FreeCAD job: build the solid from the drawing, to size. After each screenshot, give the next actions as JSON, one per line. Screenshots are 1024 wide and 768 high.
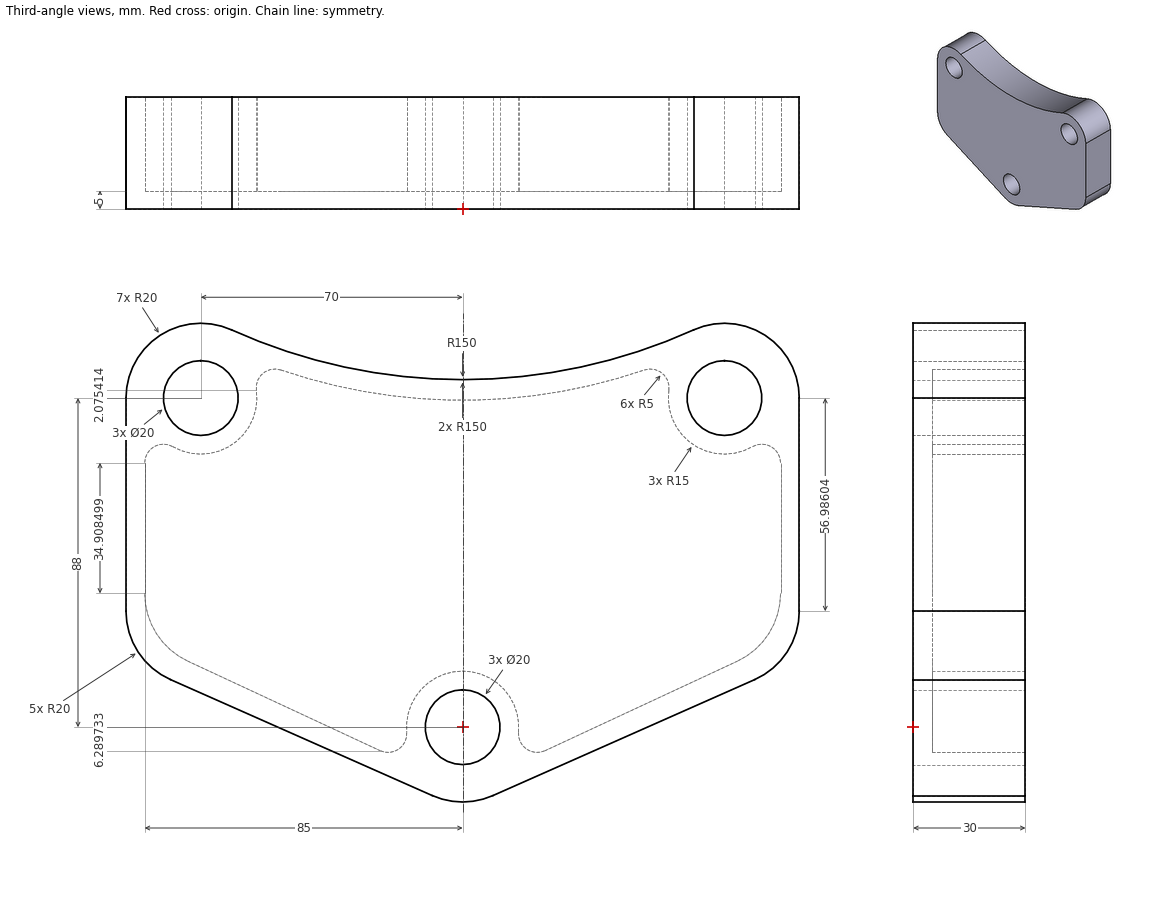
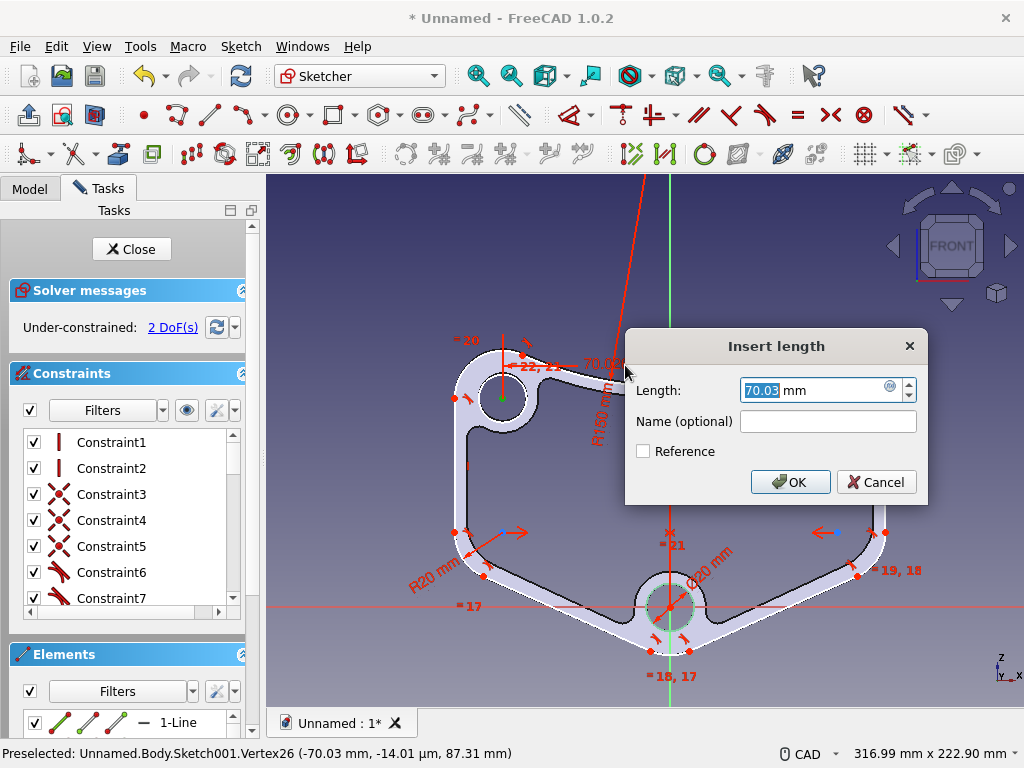
{"action": "type", "text": "70"}
{"action": "key", "text": "Return"}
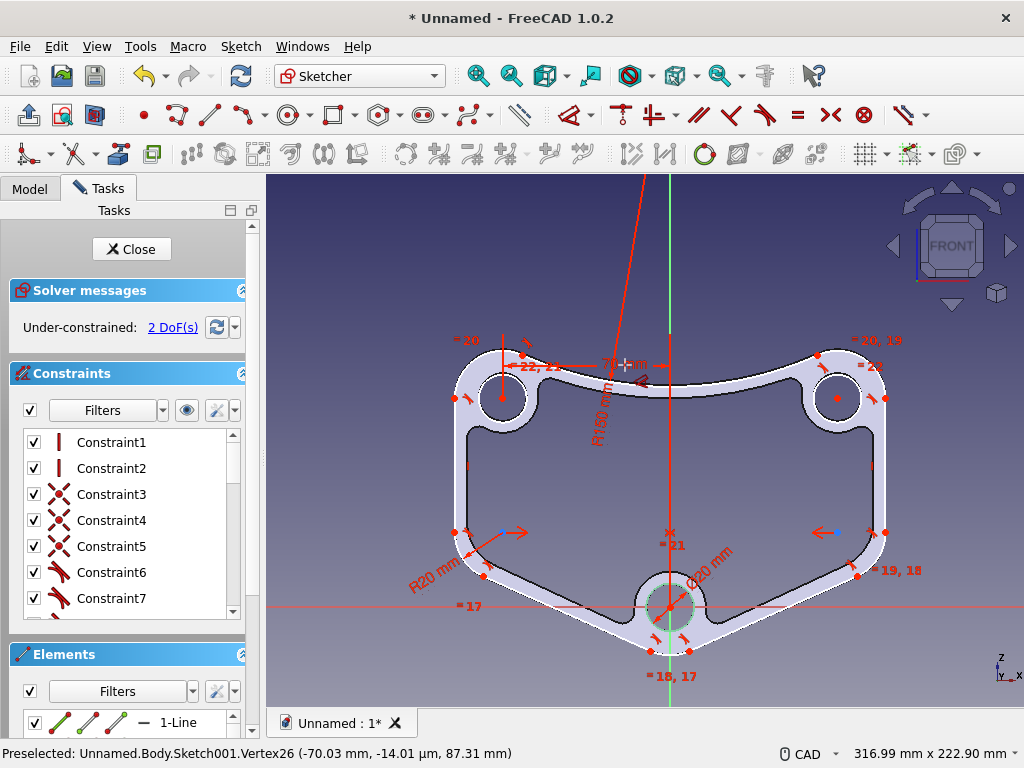
{"action": "left_click", "coordinate": [503, 399]}
{"action": "left_click", "coordinate": [469, 503]}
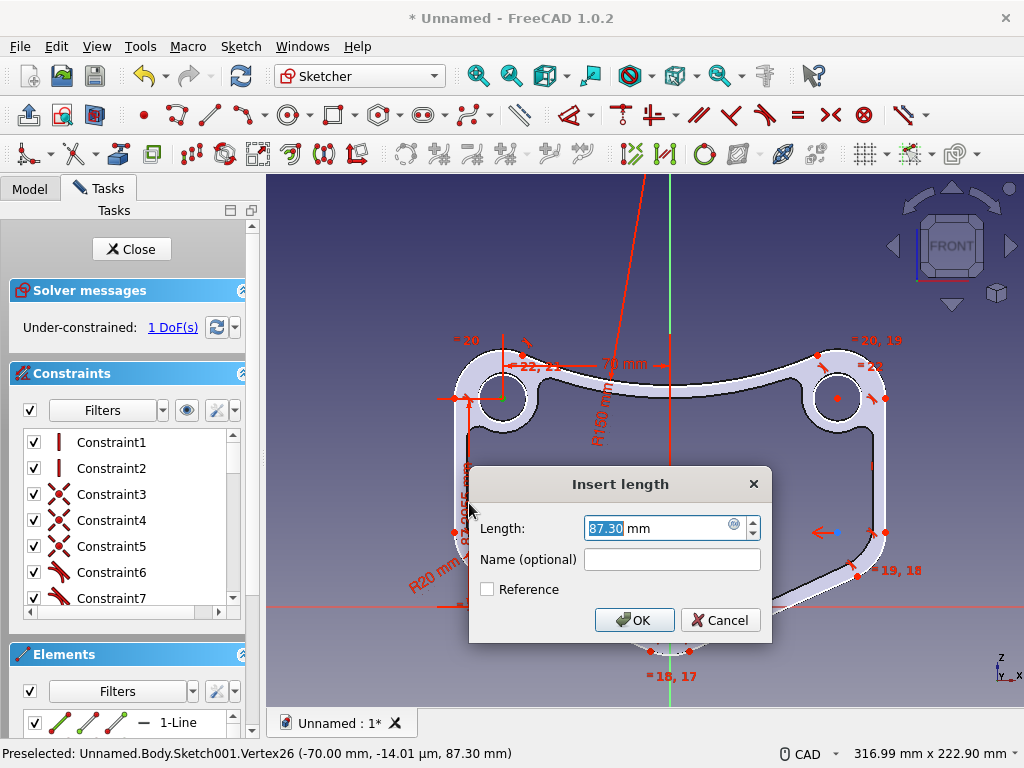
{"action": "type", "text": "88"}
{"action": "key", "text": "Return"}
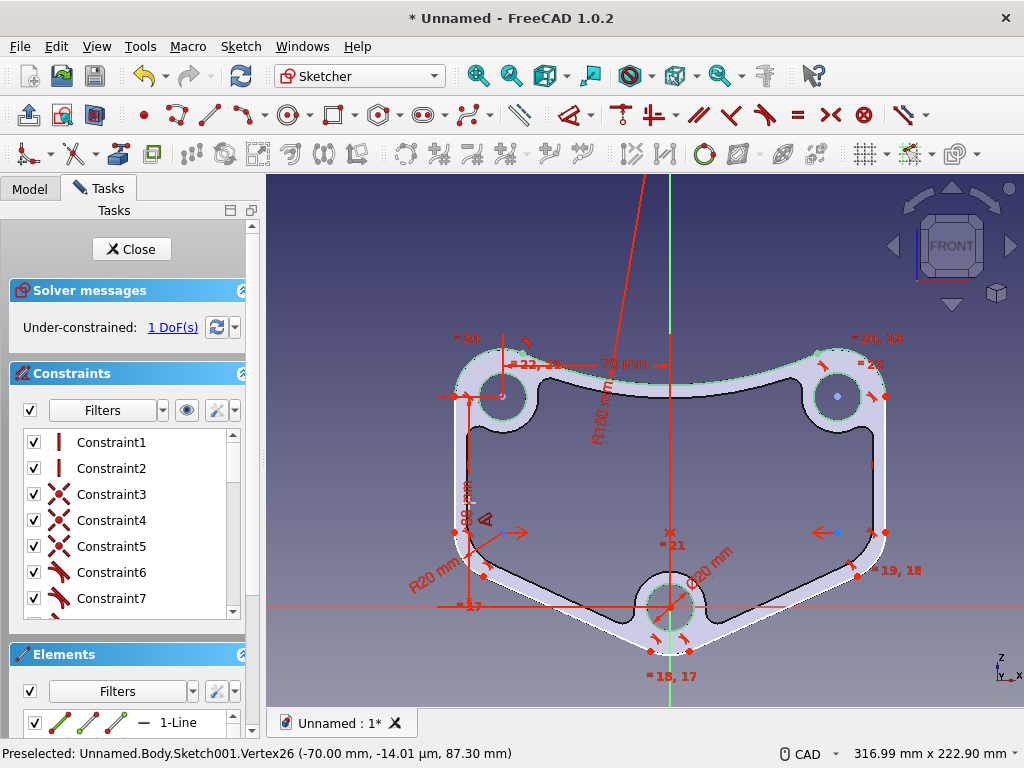
{"action": "left_click", "coordinate": [455, 438]}
{"action": "left_click", "coordinate": [421, 465]}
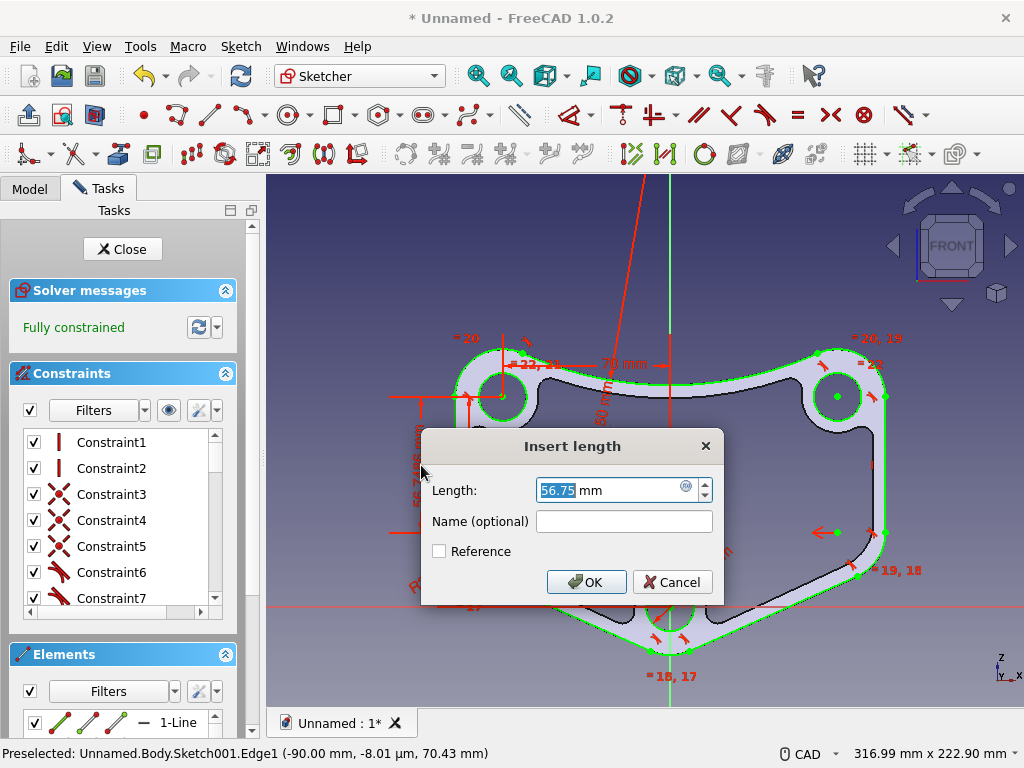
{"action": "type", "text": "56.98604"}
{"action": "key", "text": "Return"}
{"action": "key", "text": "Escape"}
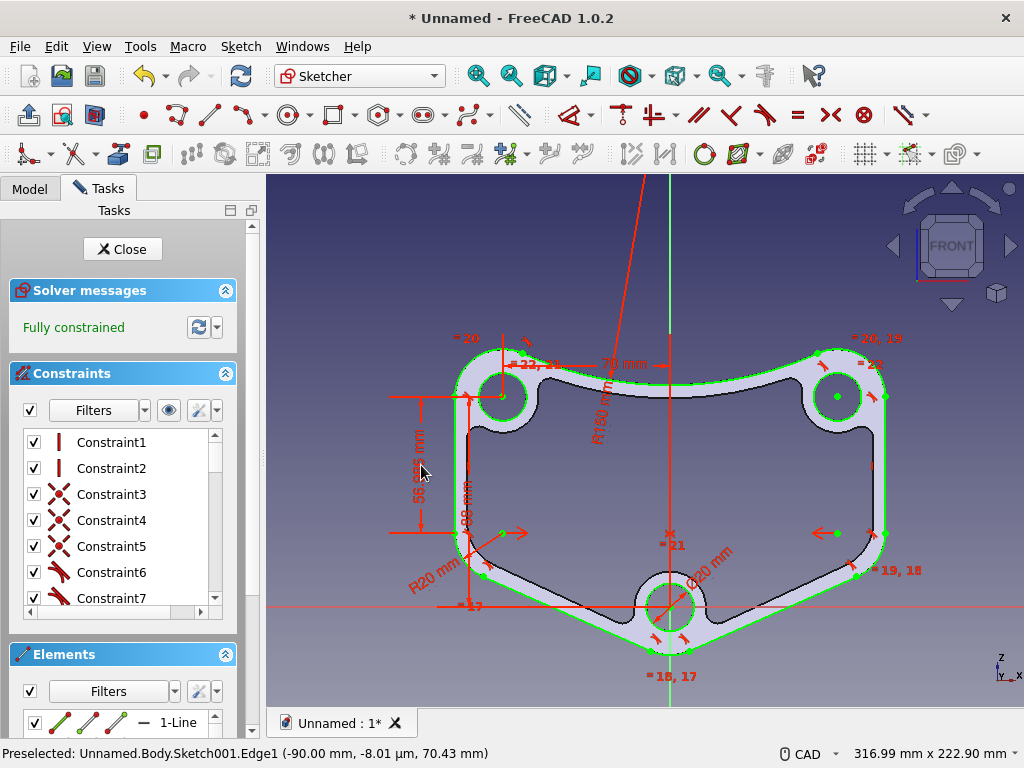
{"action": "left_click", "coordinate": [123, 249]}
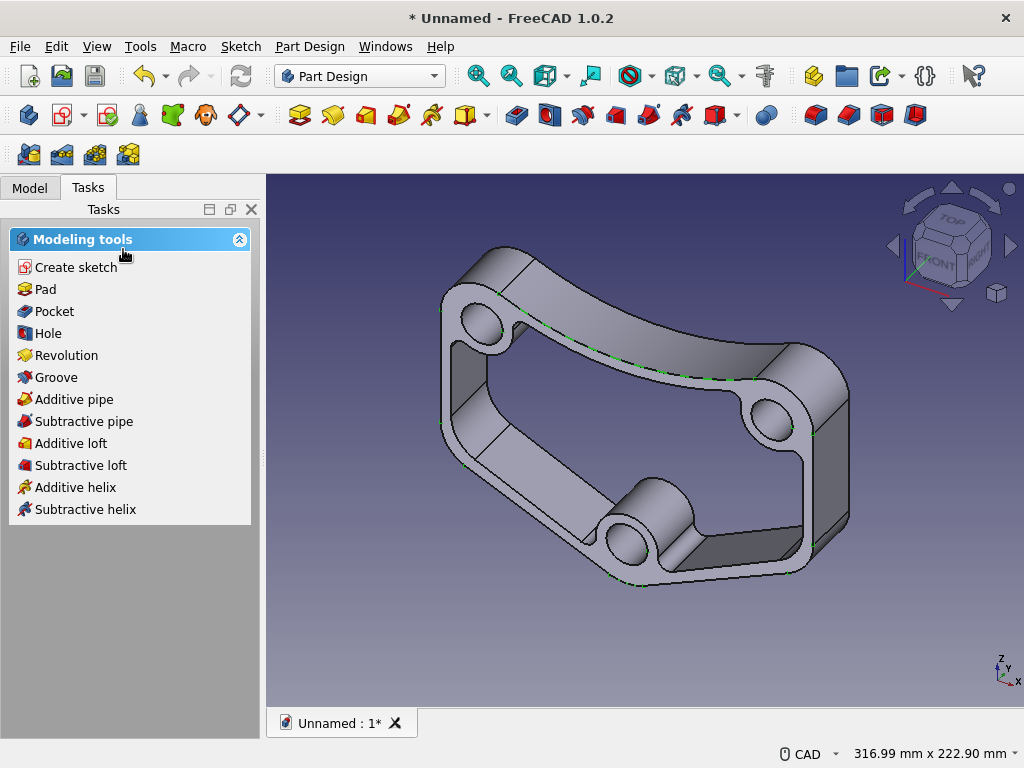
{"action": "left_click", "coordinate": [300, 116]}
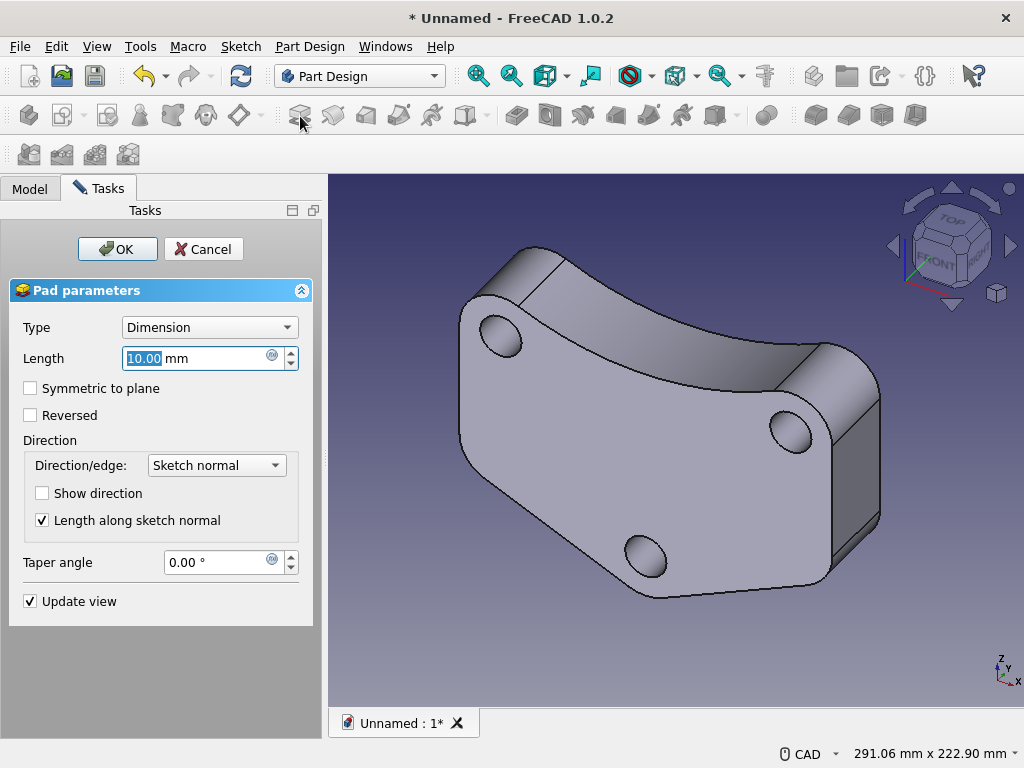
{"action": "type", "text": "5"}
{"action": "key", "text": "Tab"}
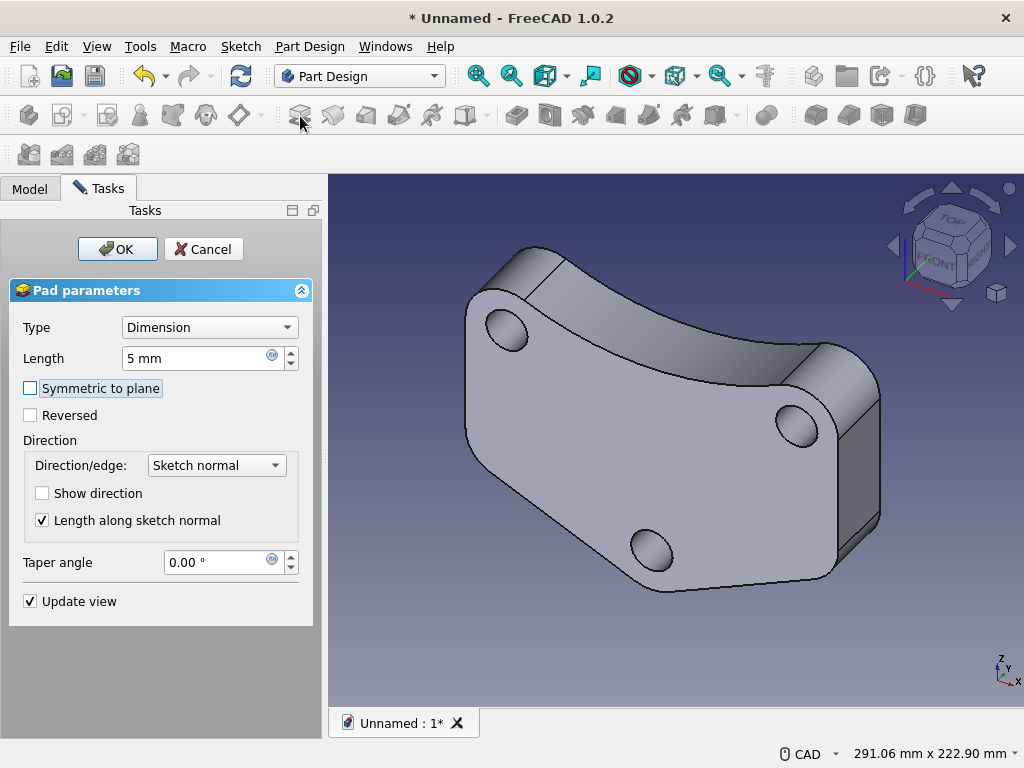
{"action": "left_click", "coordinate": [31, 415]}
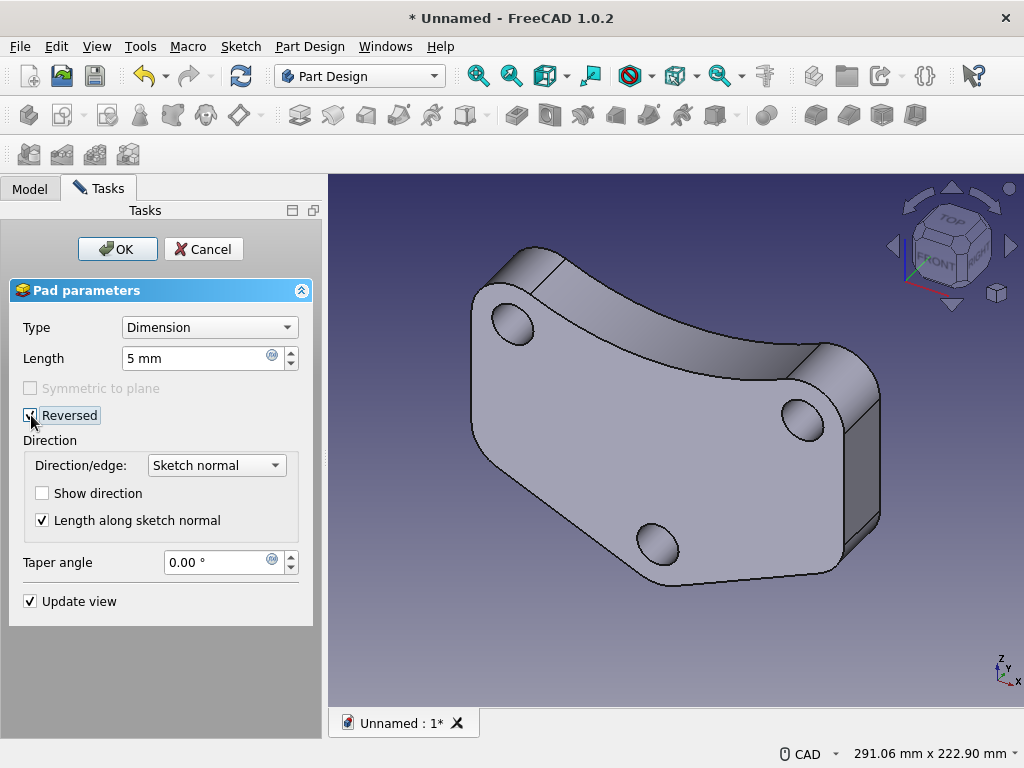
{"action": "left_click", "coordinate": [118, 249]}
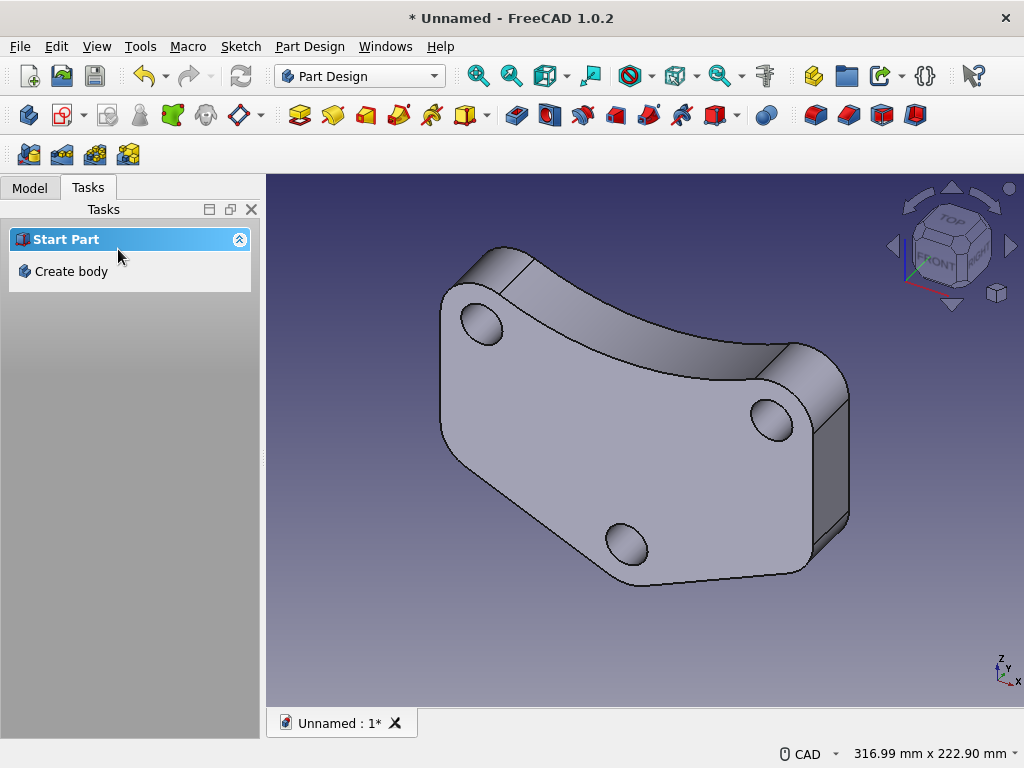
{"action": "key", "text": "0"}